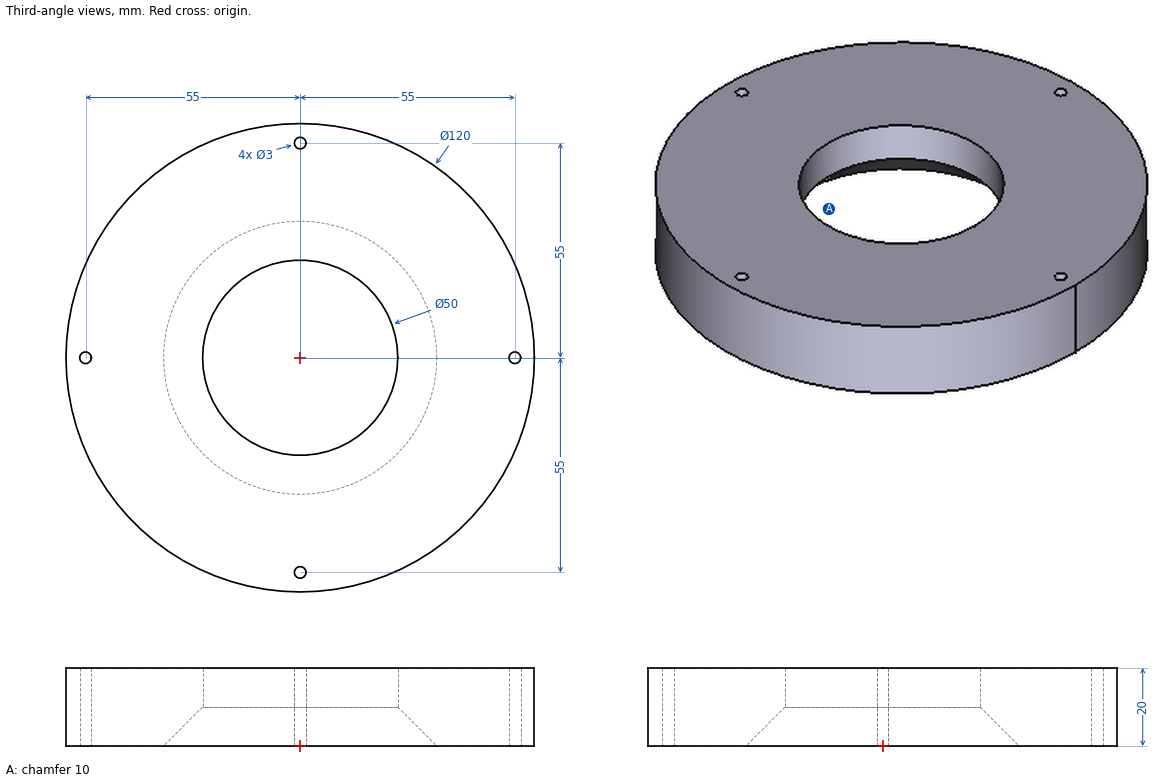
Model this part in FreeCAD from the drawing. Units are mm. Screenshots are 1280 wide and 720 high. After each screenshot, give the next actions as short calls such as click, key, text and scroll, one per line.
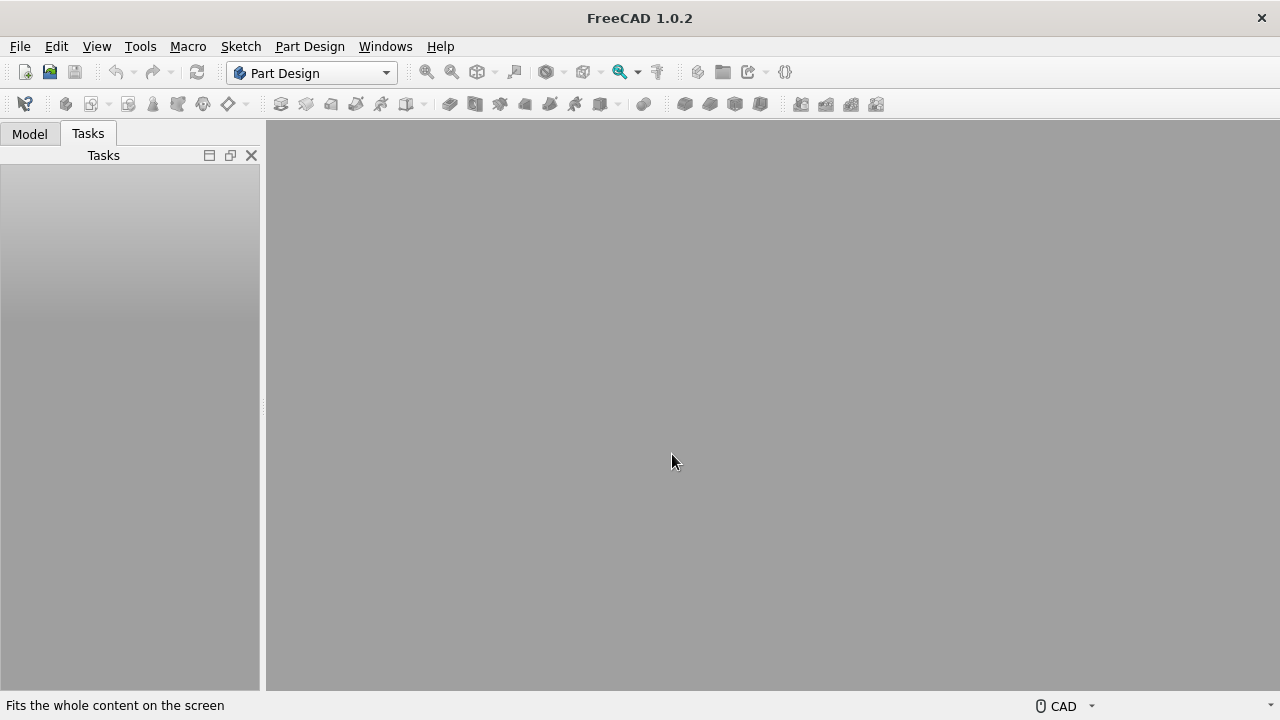
click(25, 72)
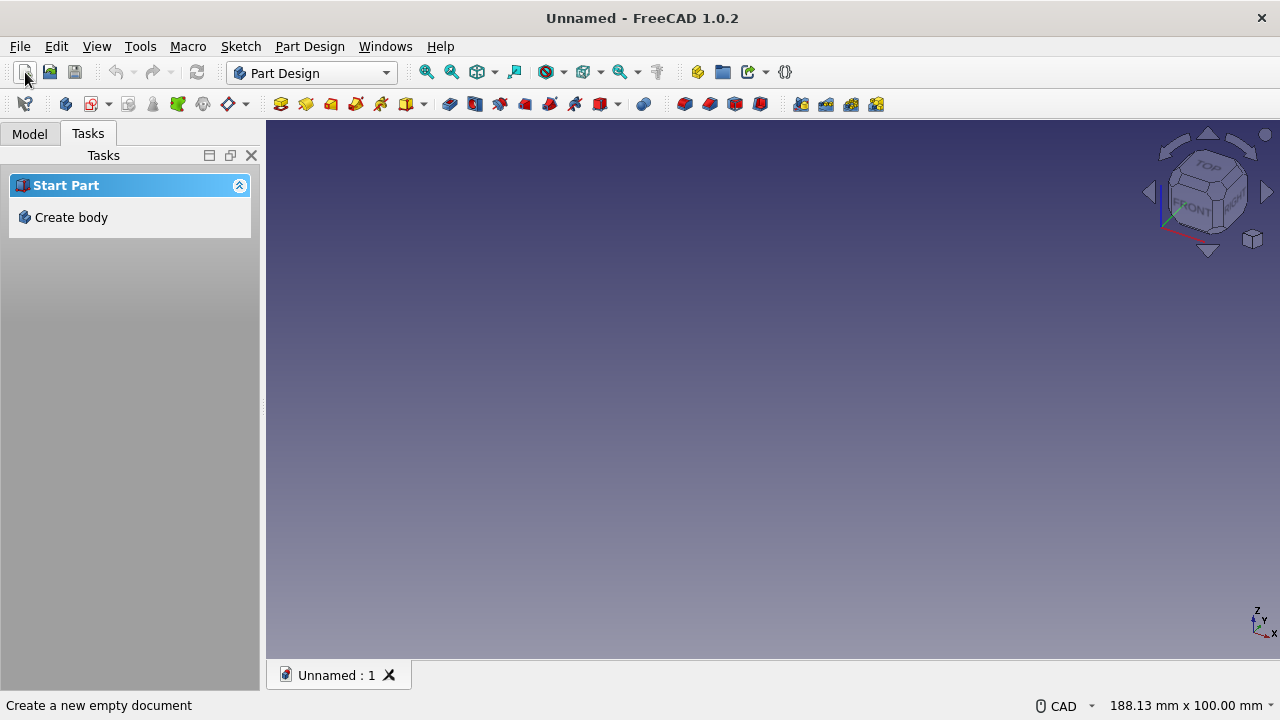
click(90, 104)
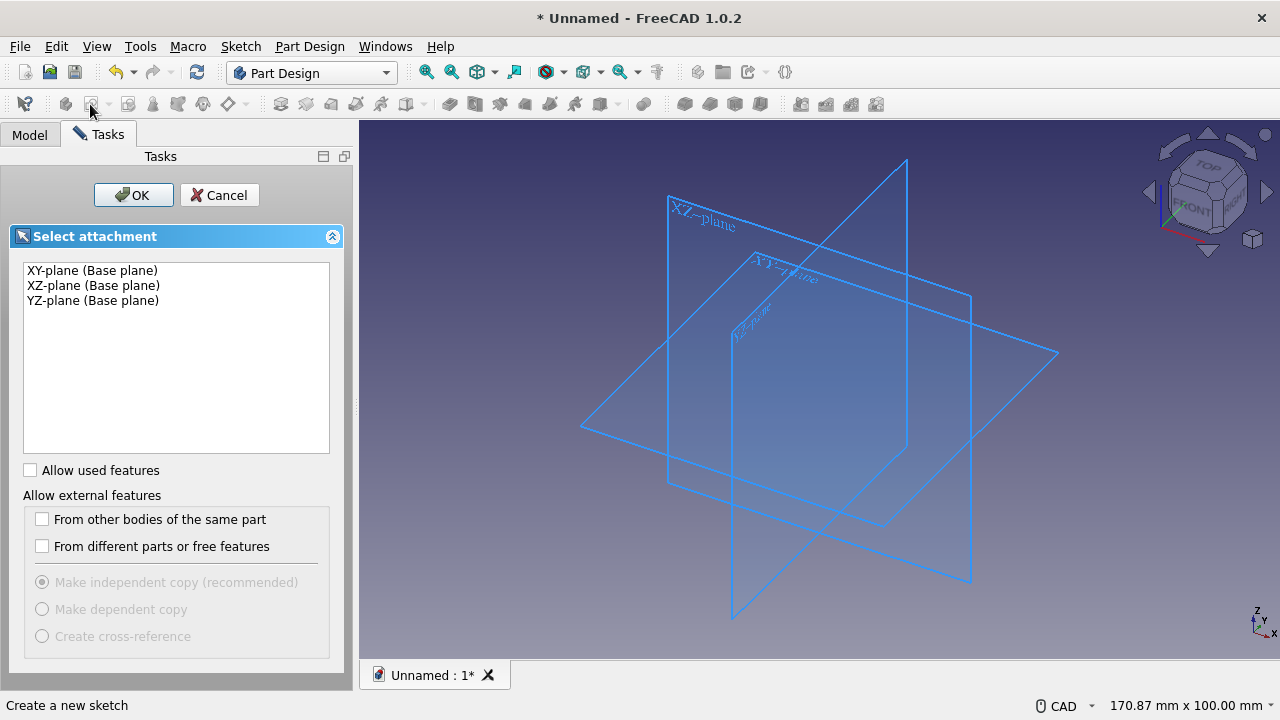
click(84, 270)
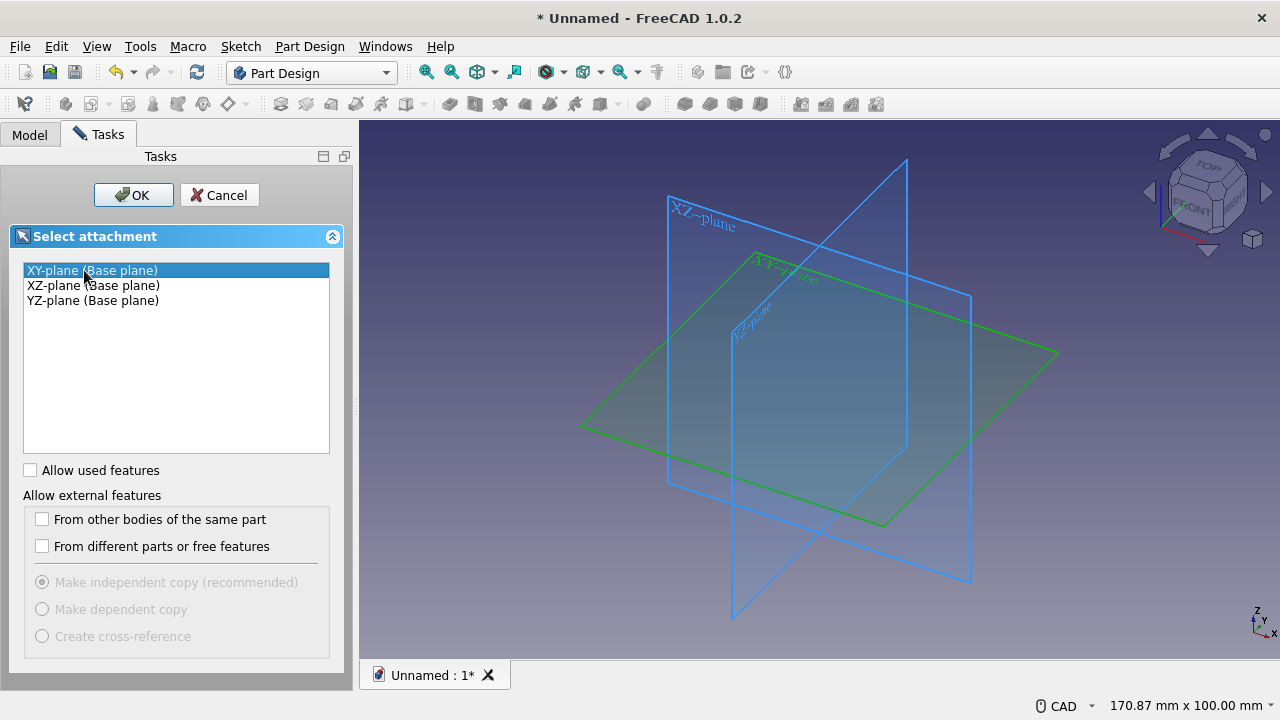
click(134, 195)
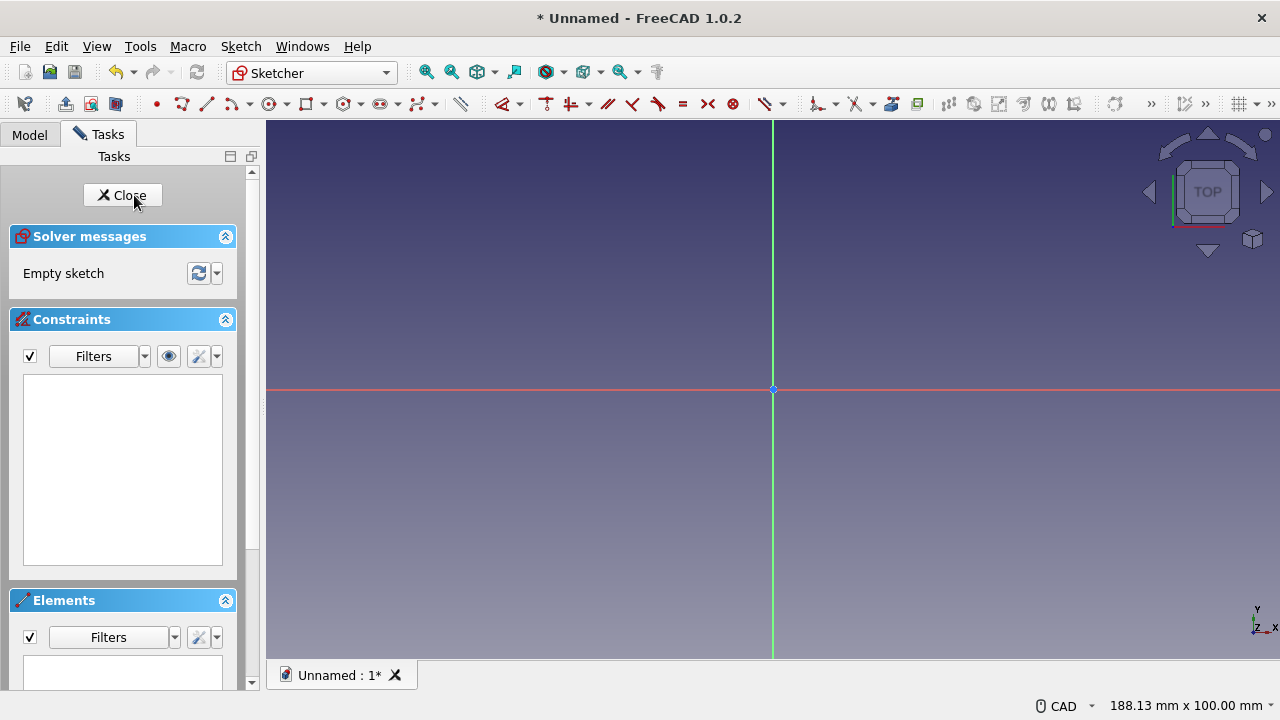
scroll(621, 390, down, 3)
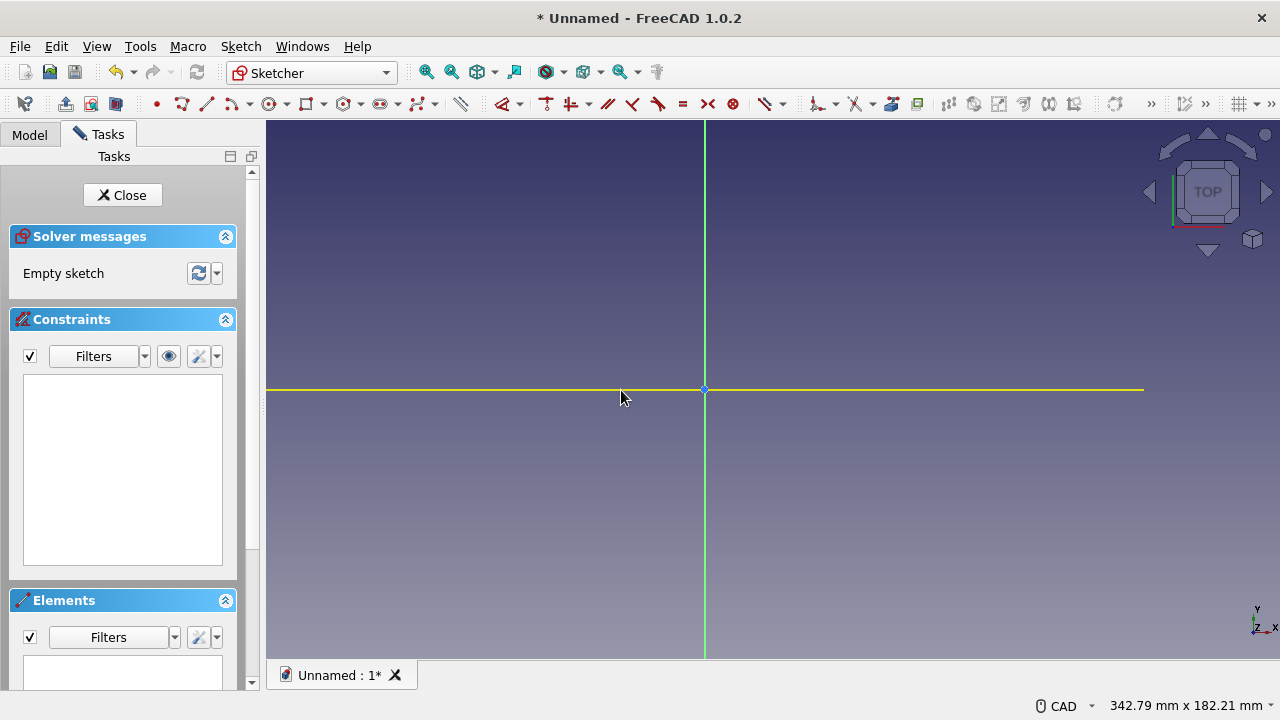
key(g)
key(c)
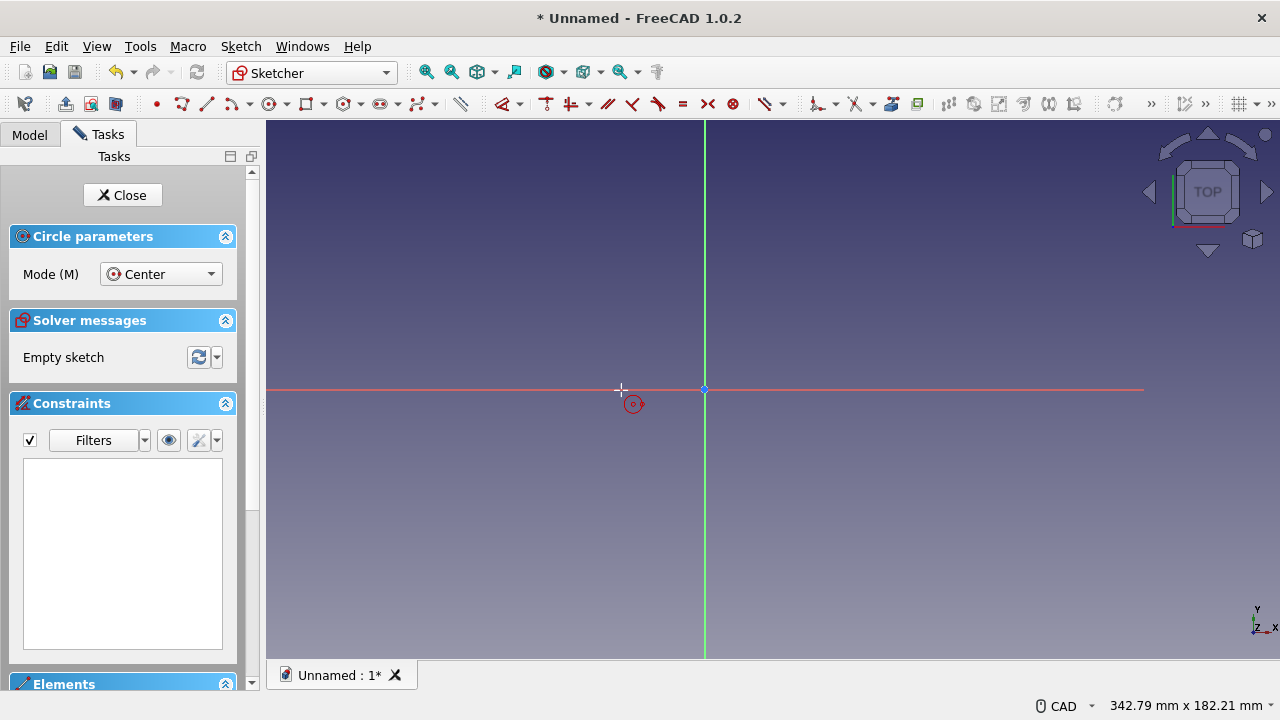
click(705, 390)
move(830, 264)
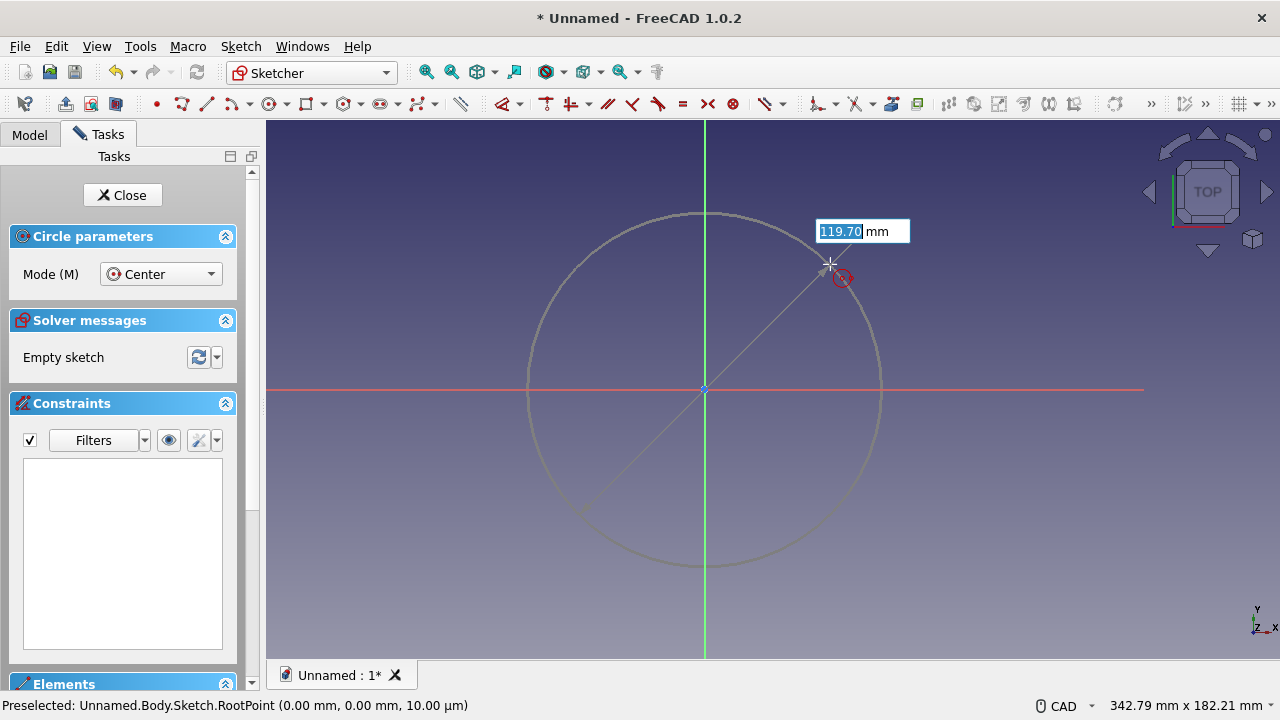
text(120)
key(Return)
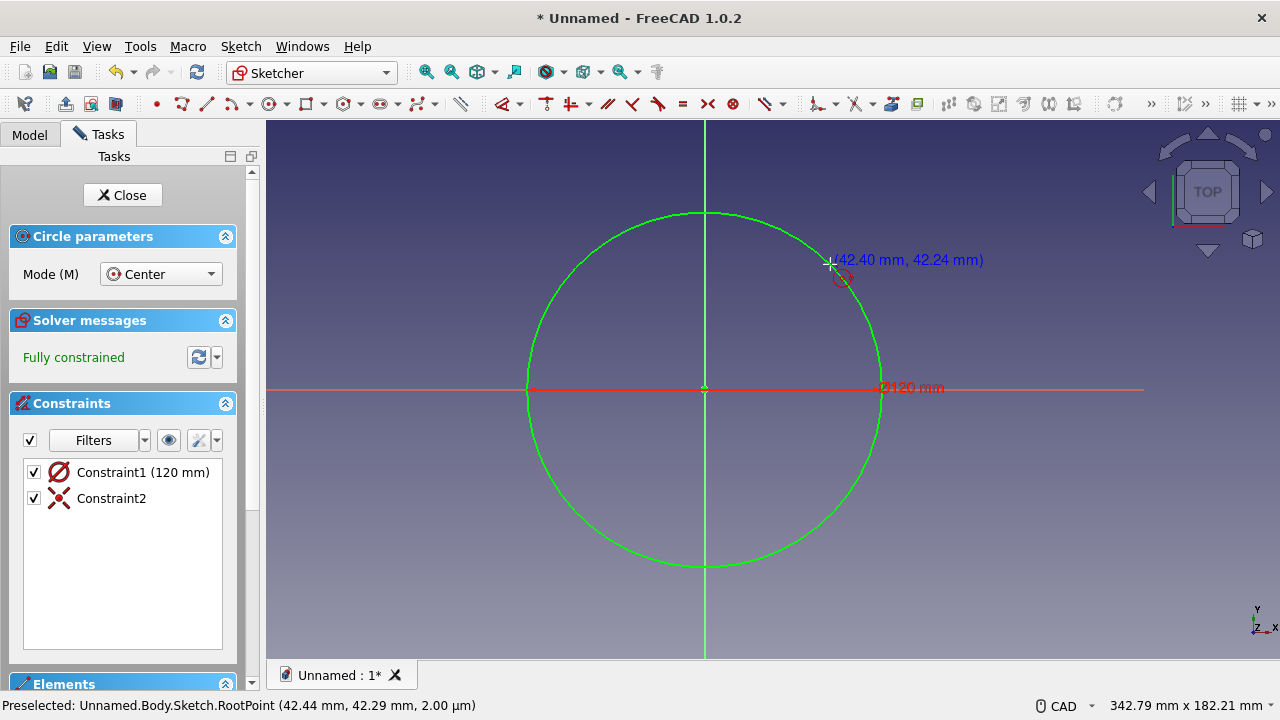
click(705, 390)
move(757, 338)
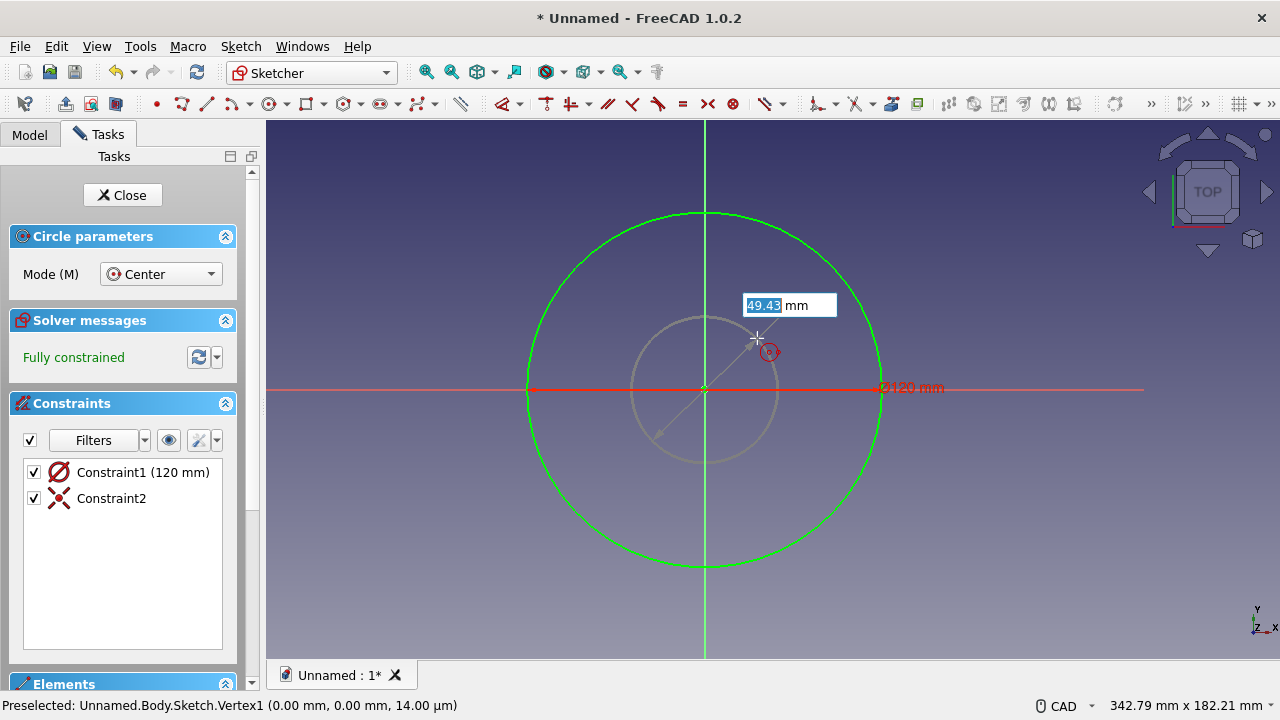
text(50)
key(Return)
key(Escape)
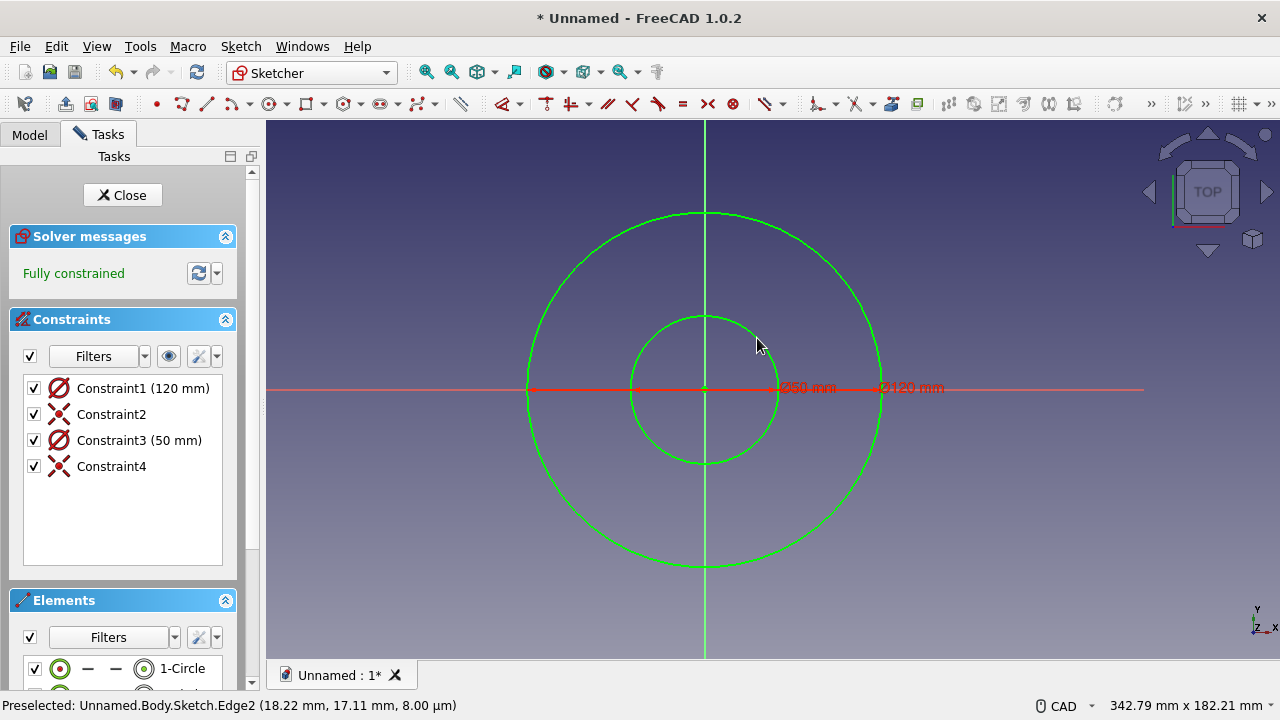
click(123, 195)